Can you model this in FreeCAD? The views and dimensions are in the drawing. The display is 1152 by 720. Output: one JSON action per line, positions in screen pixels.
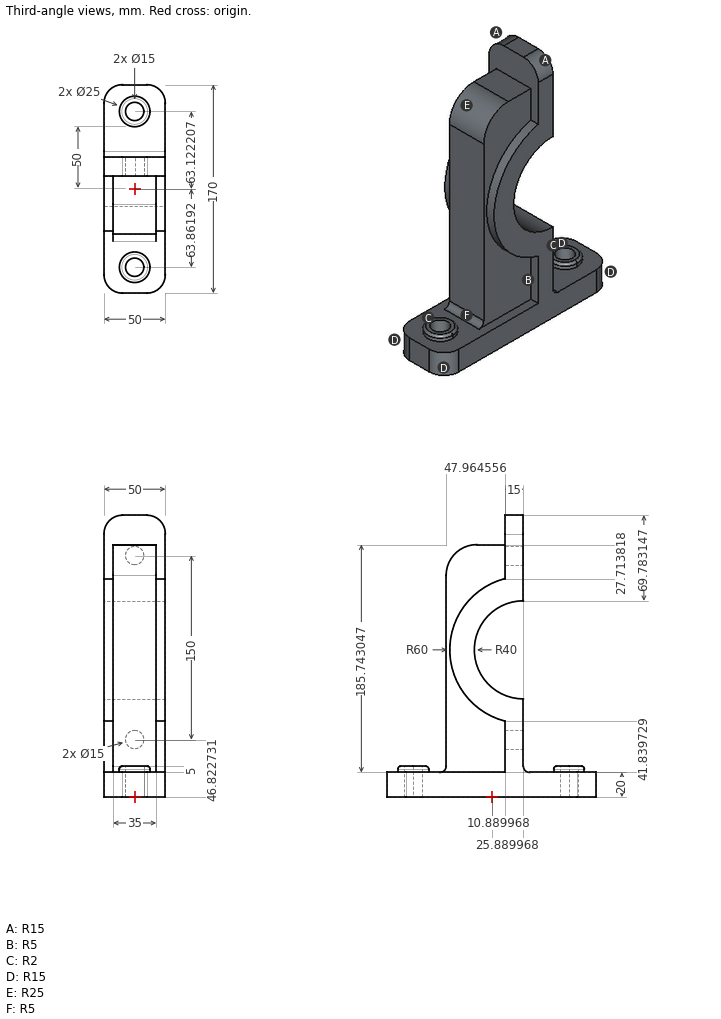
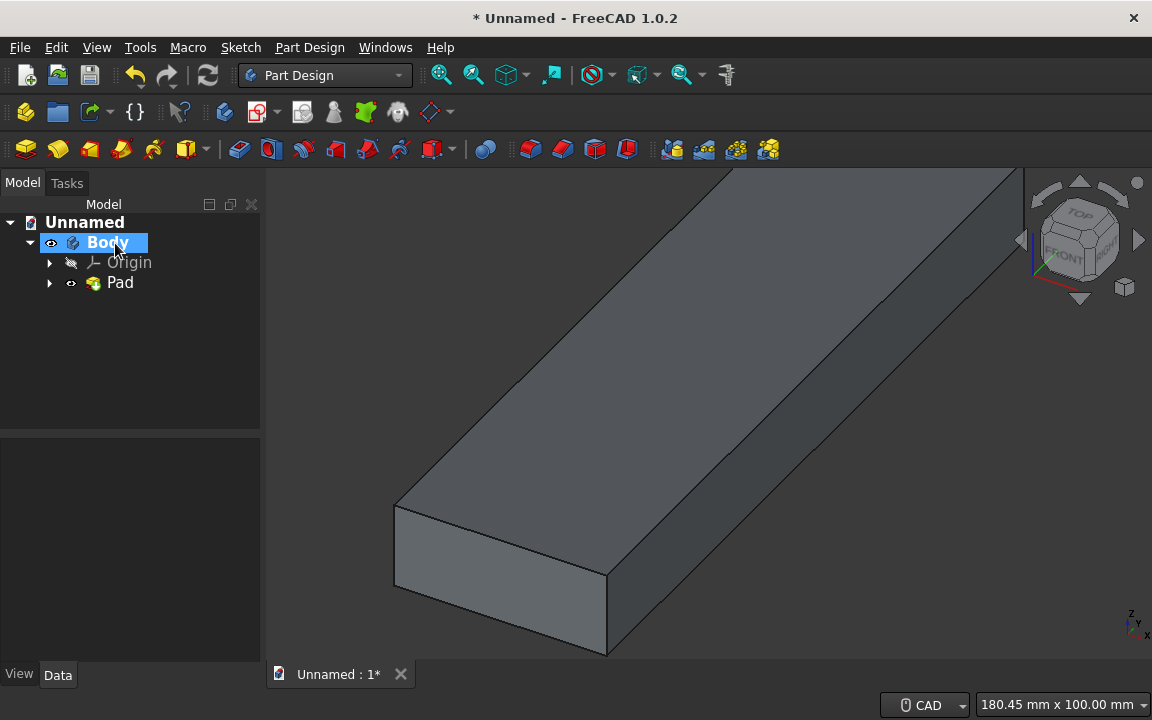
{"action": "key", "text": "v f"}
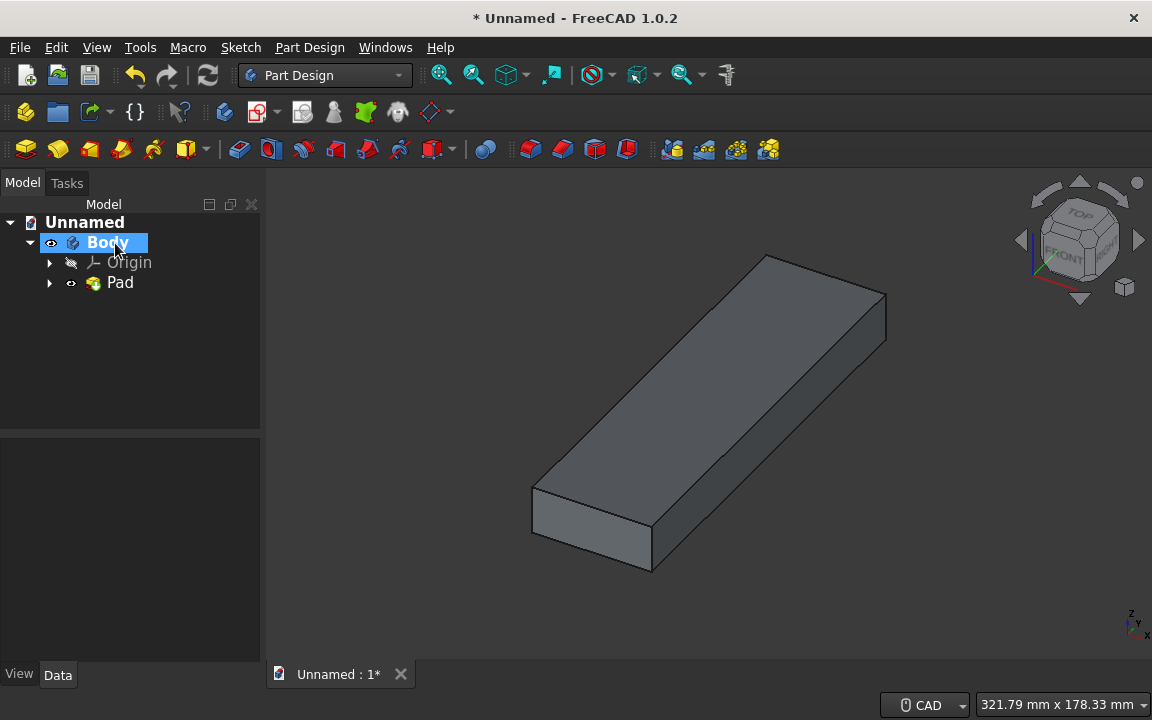
{"action": "left_click", "coordinate": [258, 112]}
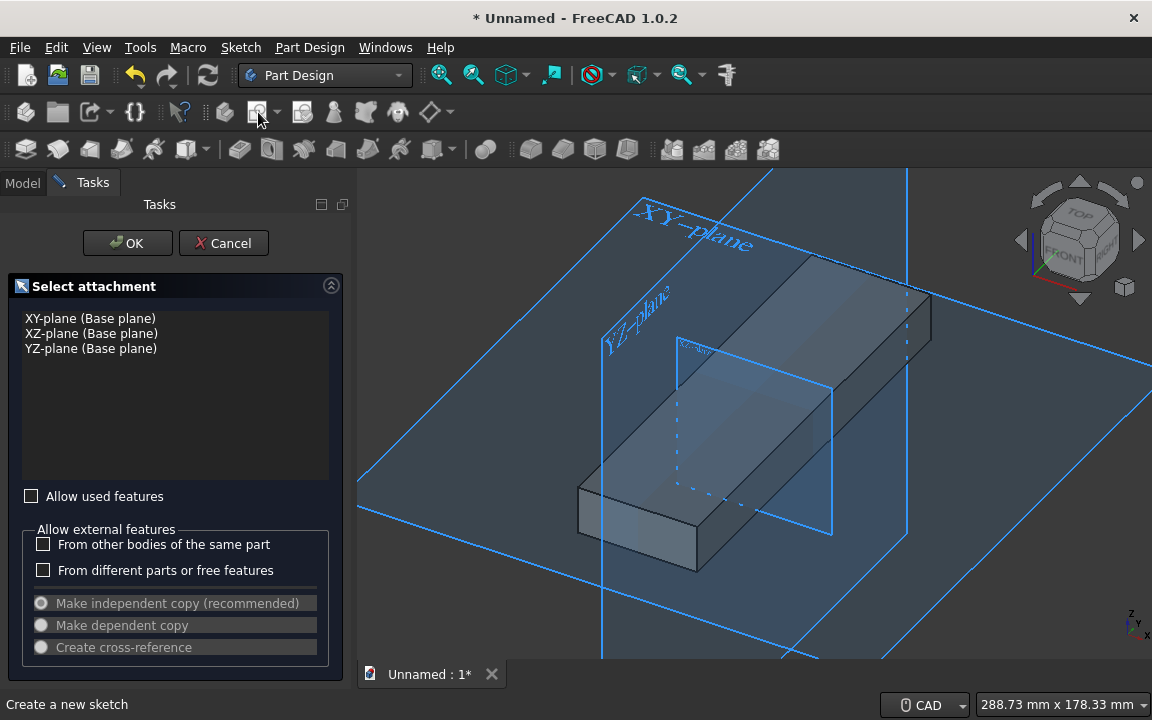
{"action": "left_click", "coordinate": [82, 348]}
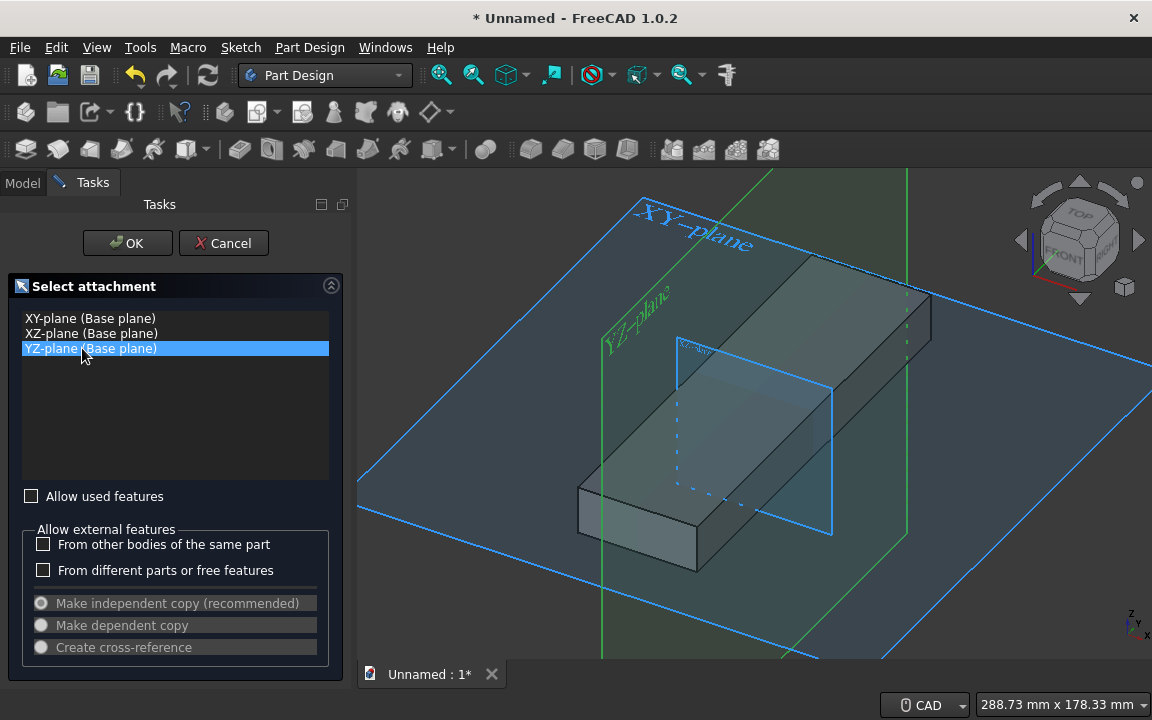
{"action": "left_click", "coordinate": [128, 243]}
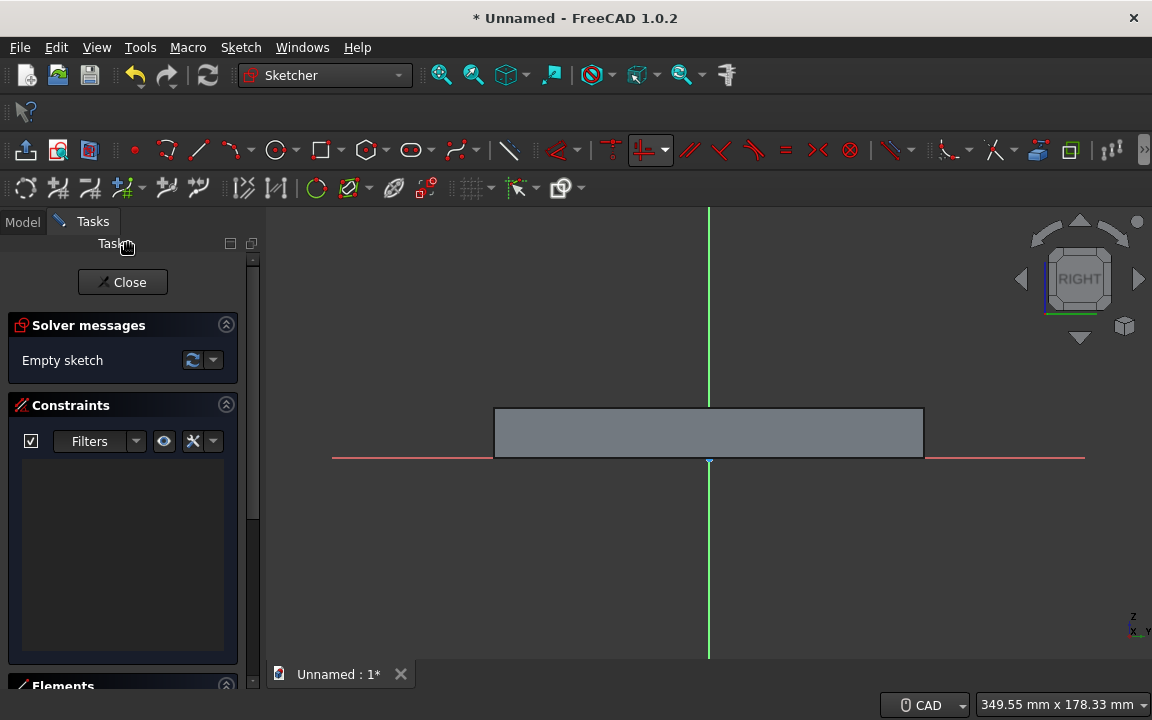
{"action": "key", "text": "q s"}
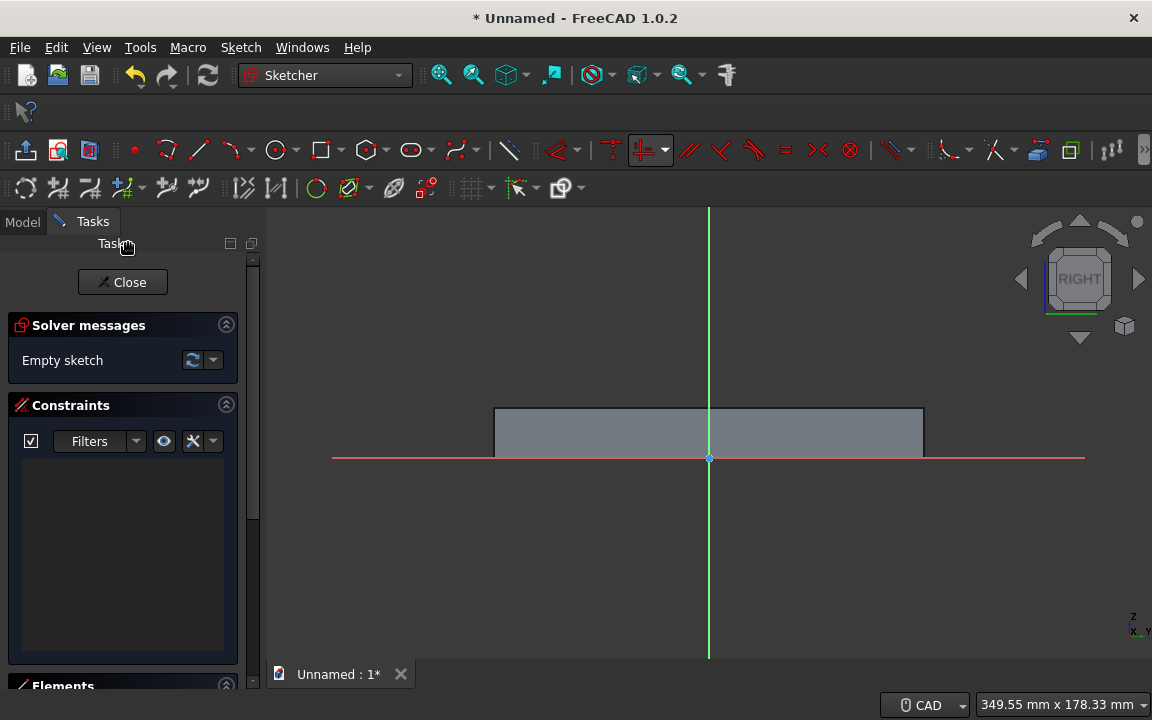
{"action": "scroll", "coordinate": [593, 631], "scroll_direction": "down", "scroll_amount": 4}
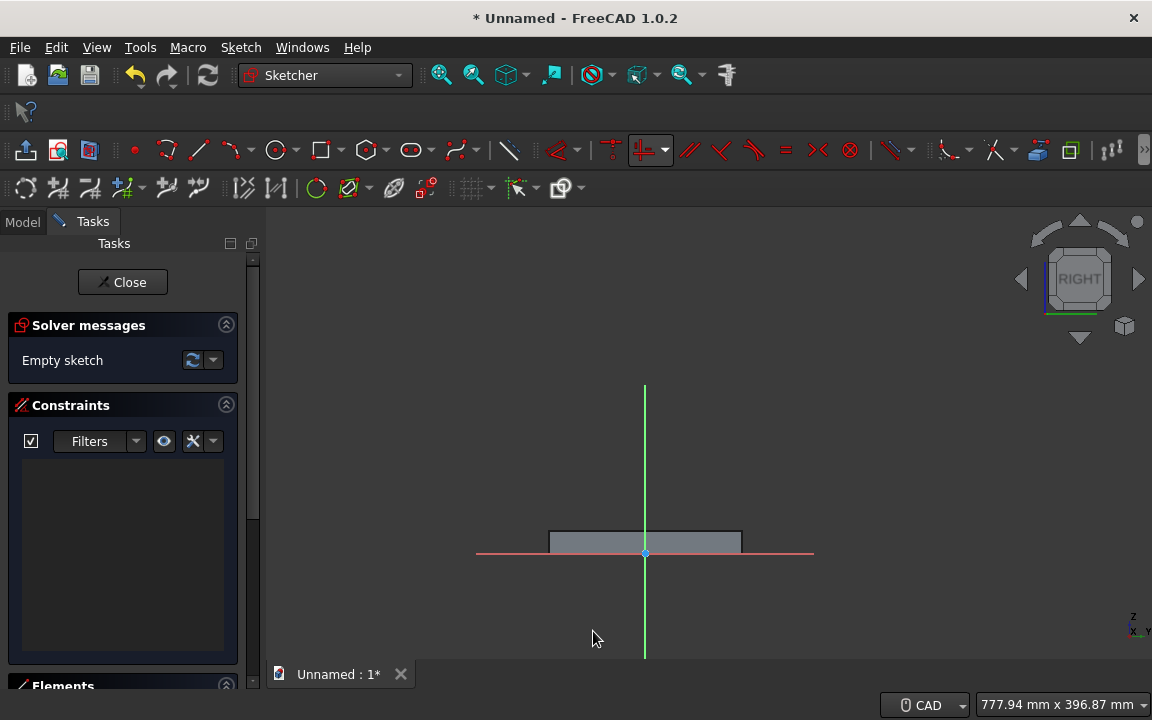
{"action": "left_click", "coordinate": [168, 150]}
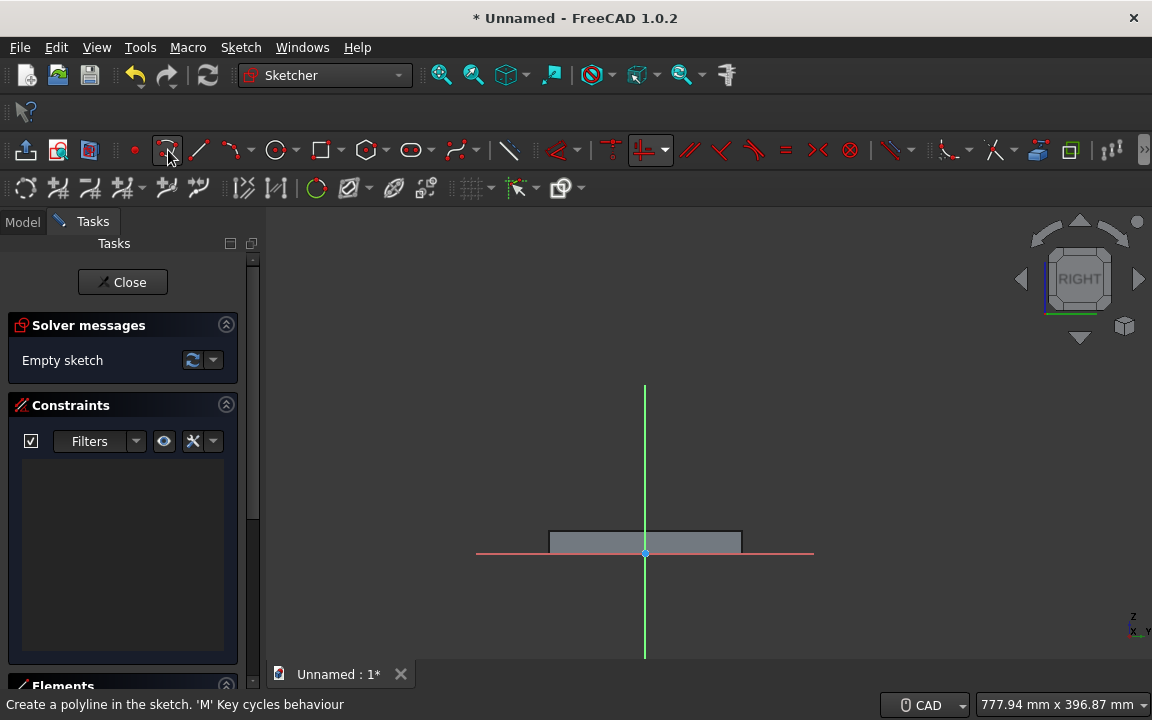
{"action": "left_click", "coordinate": [675, 372]}
{"action": "left_click", "coordinate": [675, 292]}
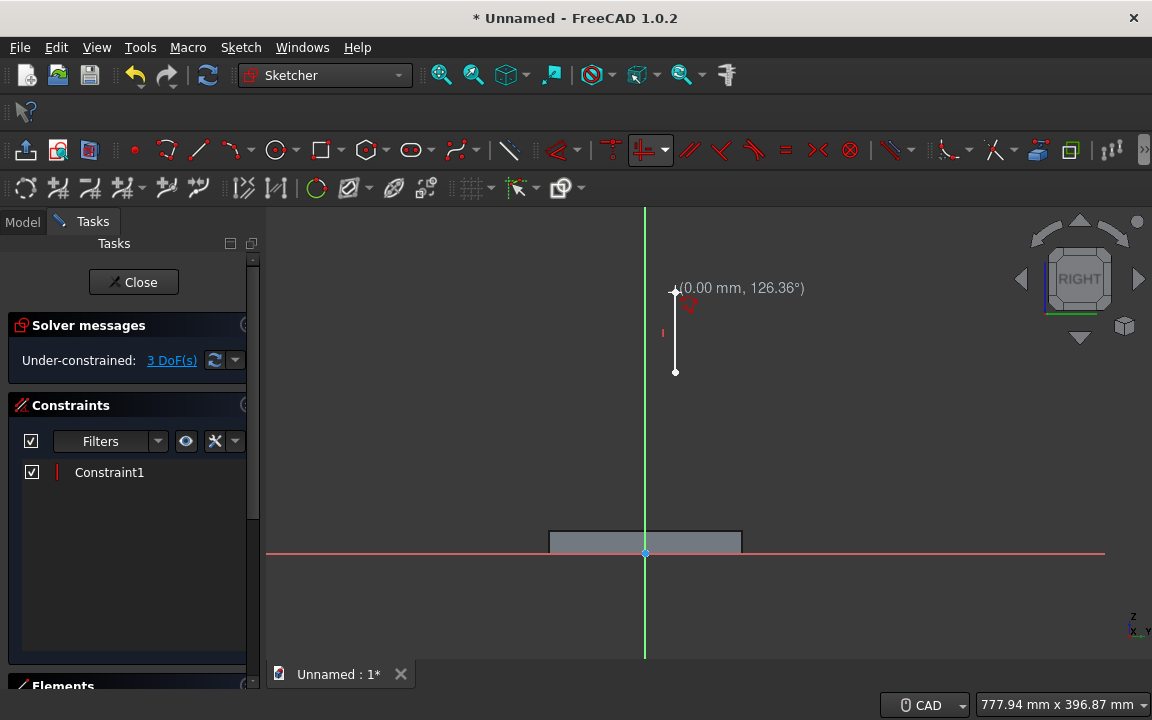
{"action": "scroll", "coordinate": [658, 292], "scroll_direction": "up", "scroll_amount": 2}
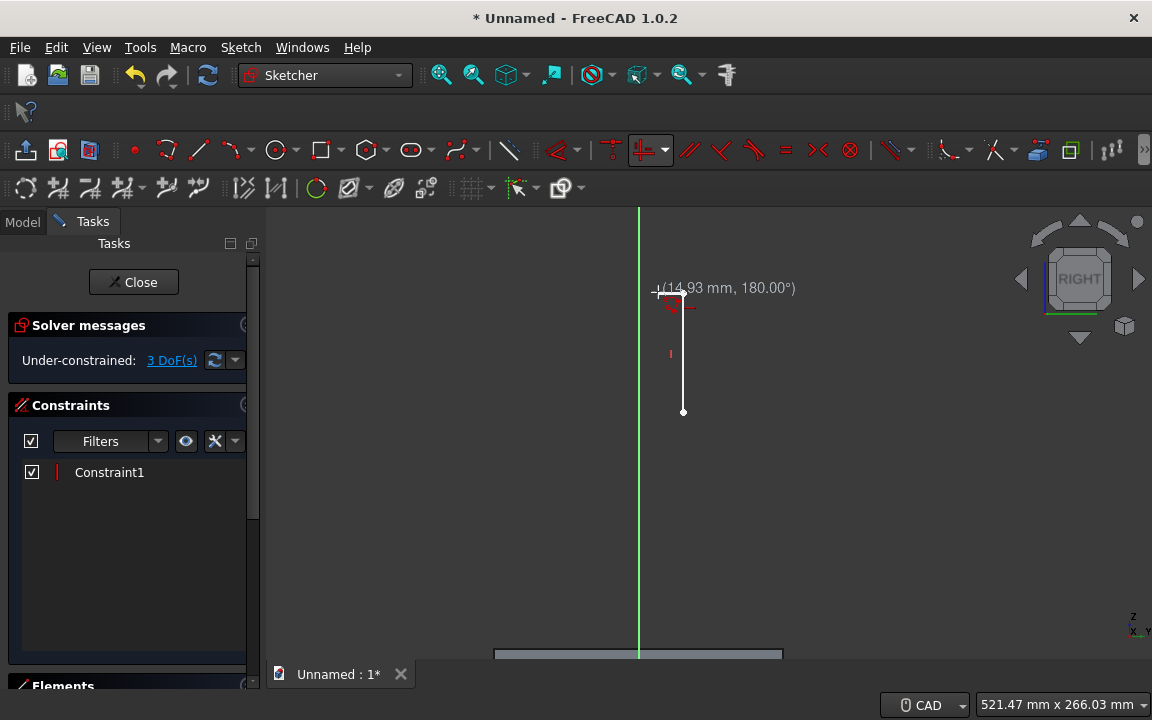
{"action": "left_click", "coordinate": [657, 292]}
{"action": "left_click", "coordinate": [657, 380]}
{"action": "right_click", "coordinate": [657, 380]}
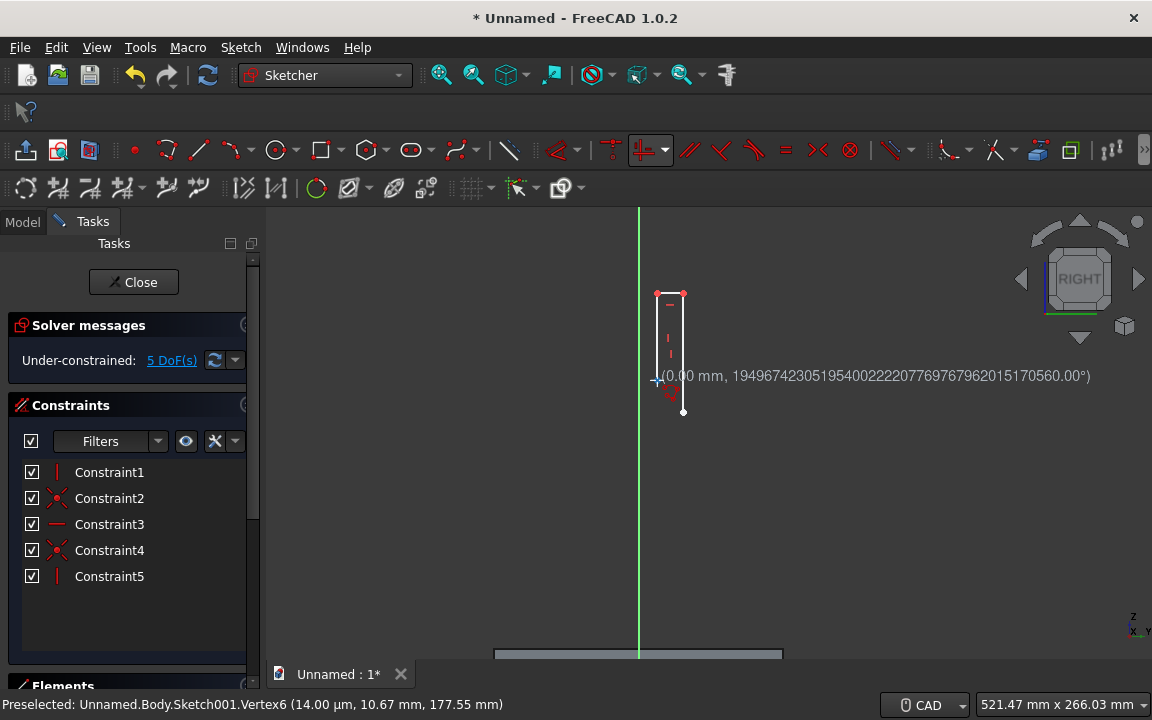
{"action": "left_click", "coordinate": [657, 578]}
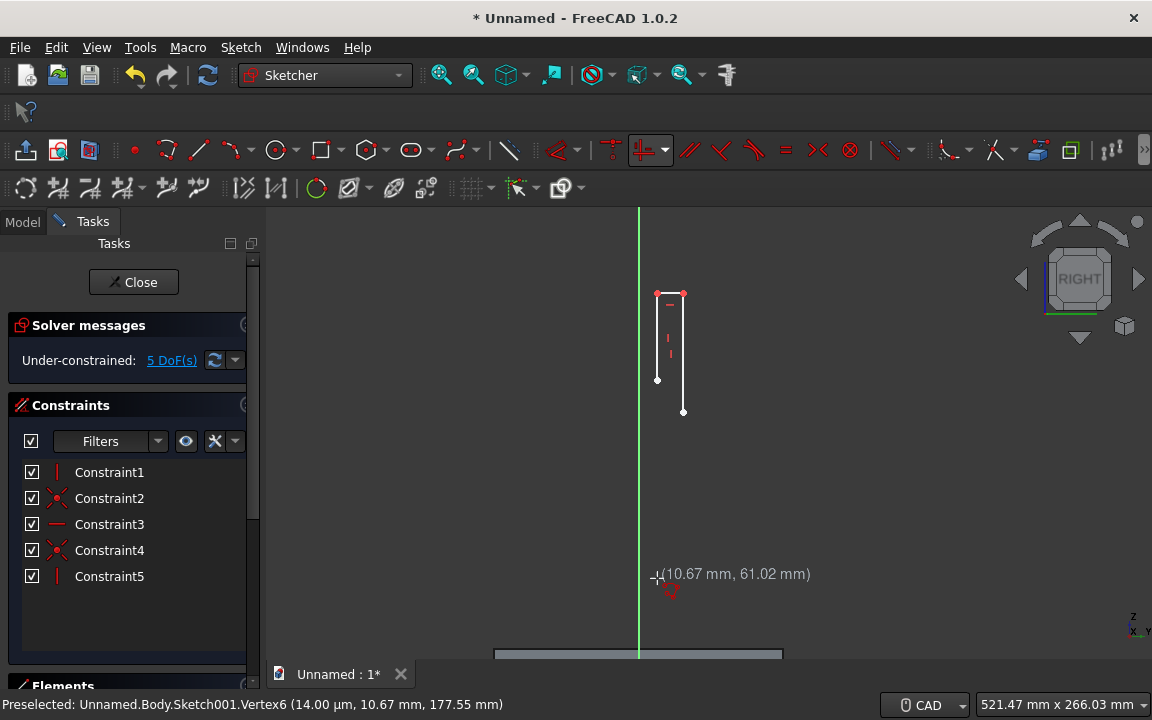
{"action": "scroll", "coordinate": [658, 322], "scroll_direction": "down", "scroll_amount": 2}